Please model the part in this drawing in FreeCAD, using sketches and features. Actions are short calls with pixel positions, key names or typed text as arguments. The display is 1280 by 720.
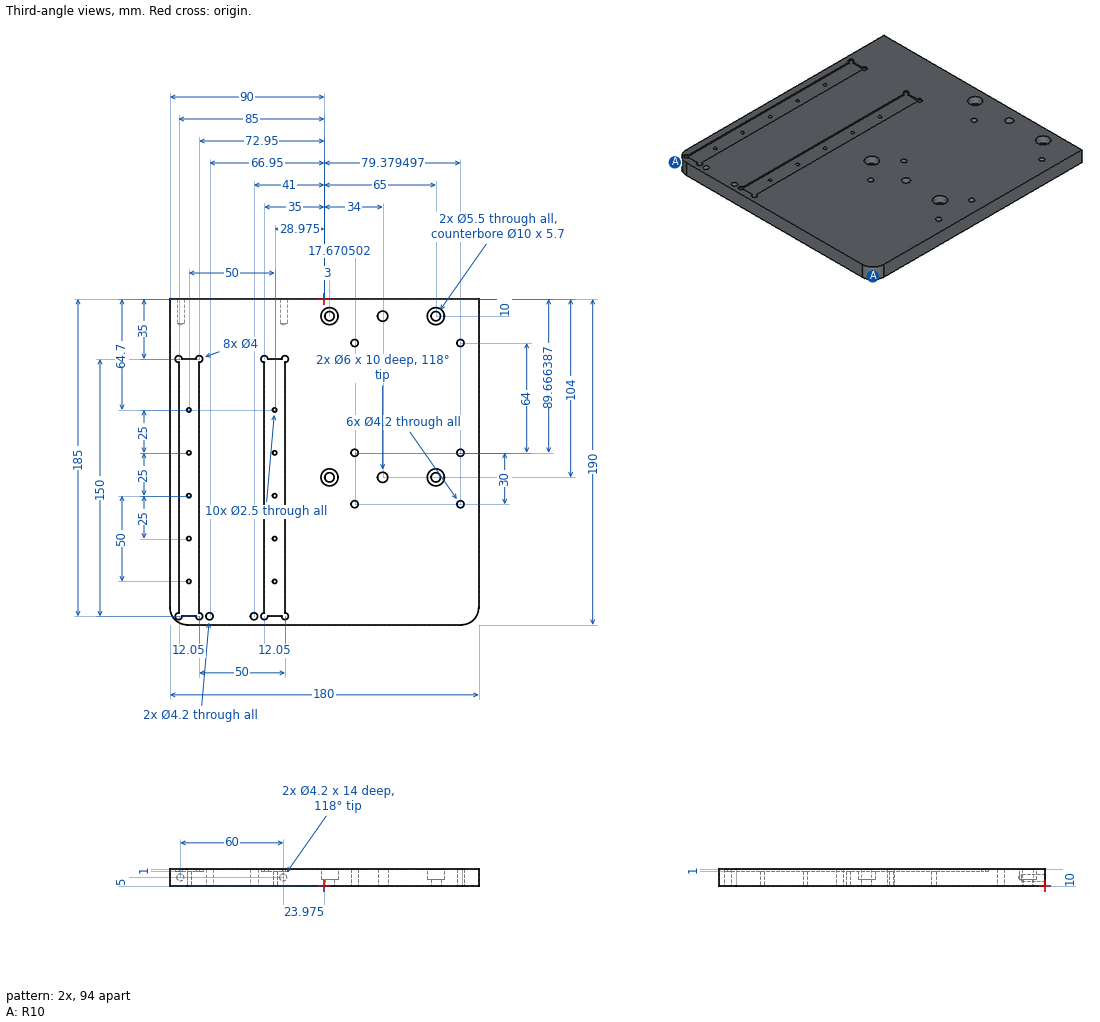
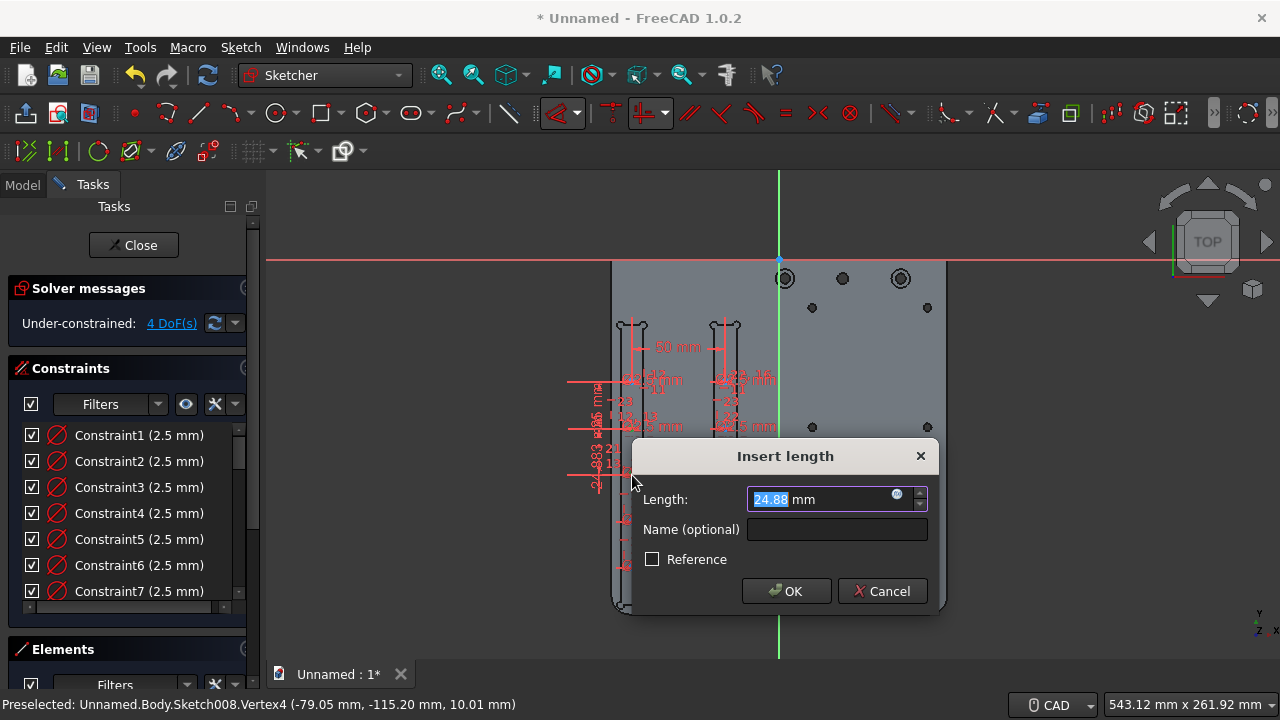
text(25)
key(Return)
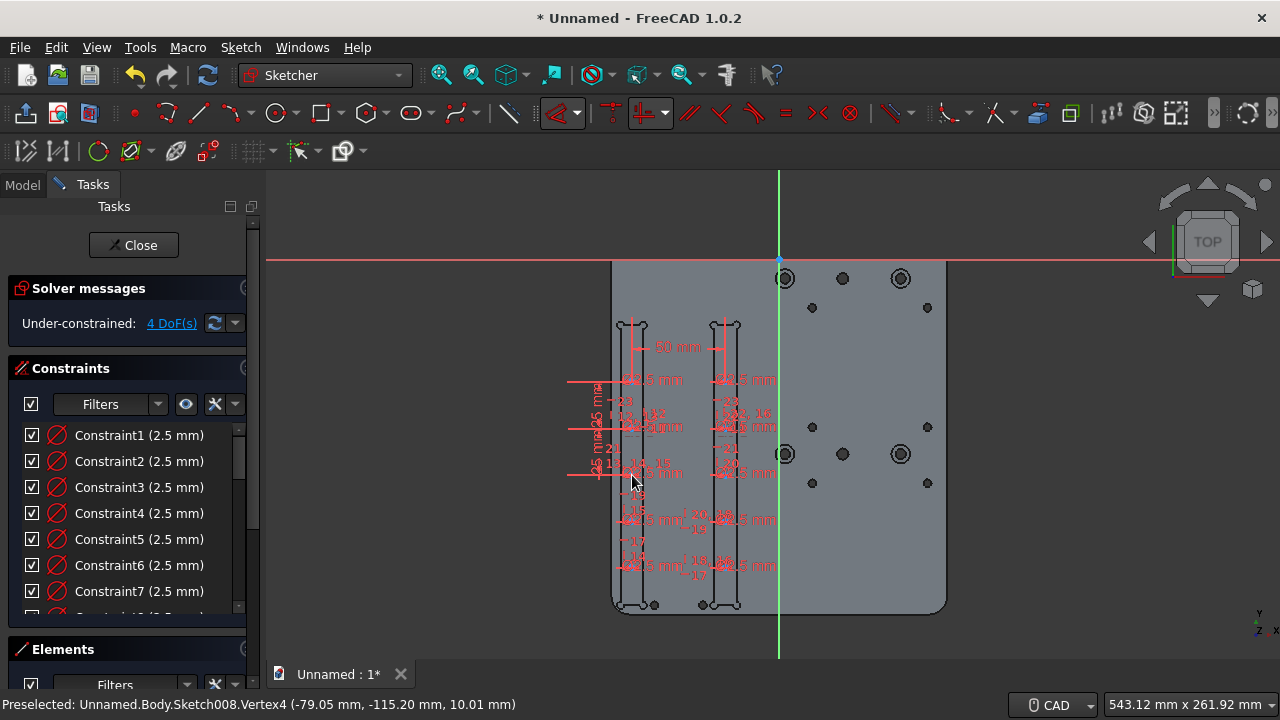
click(632, 475)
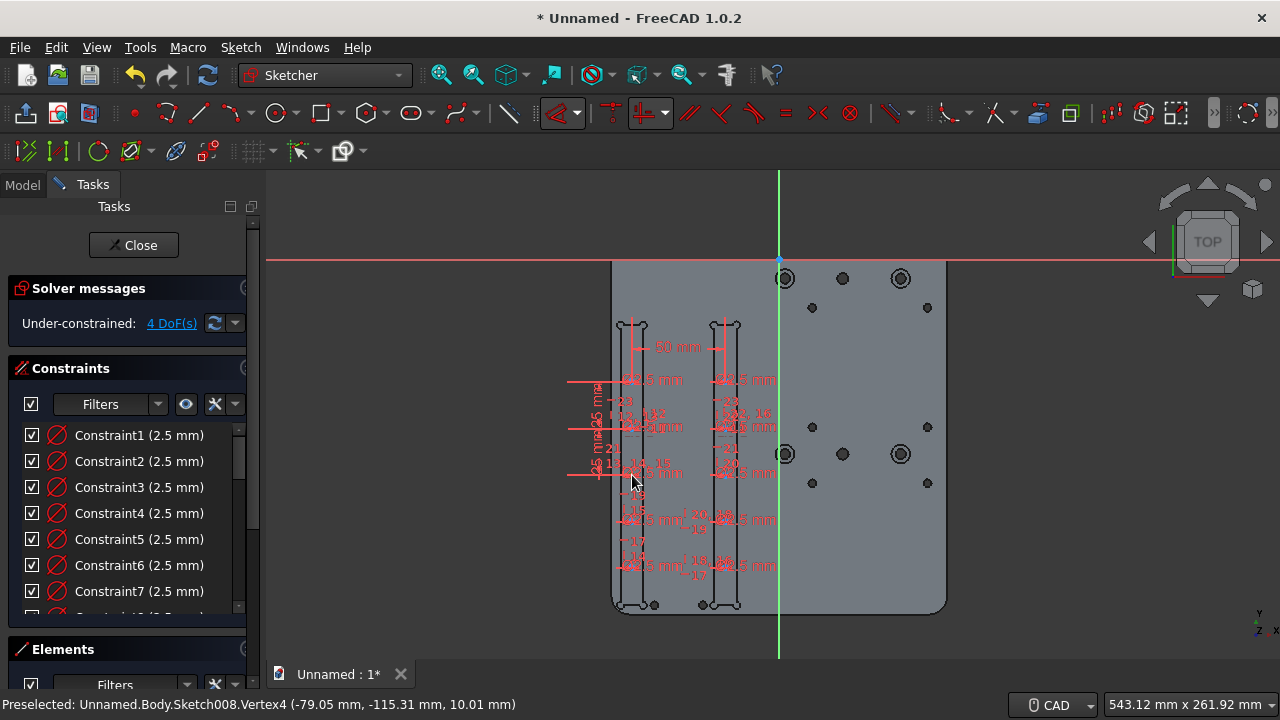
click(632, 568)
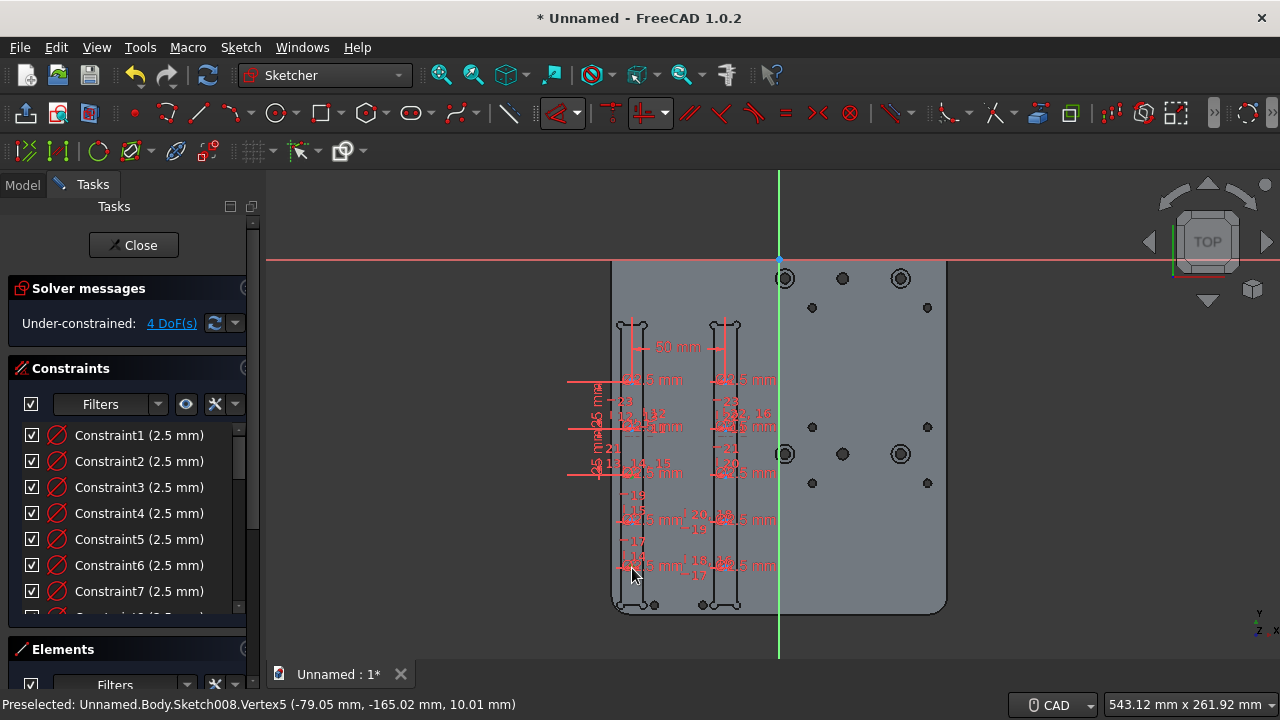
key(i)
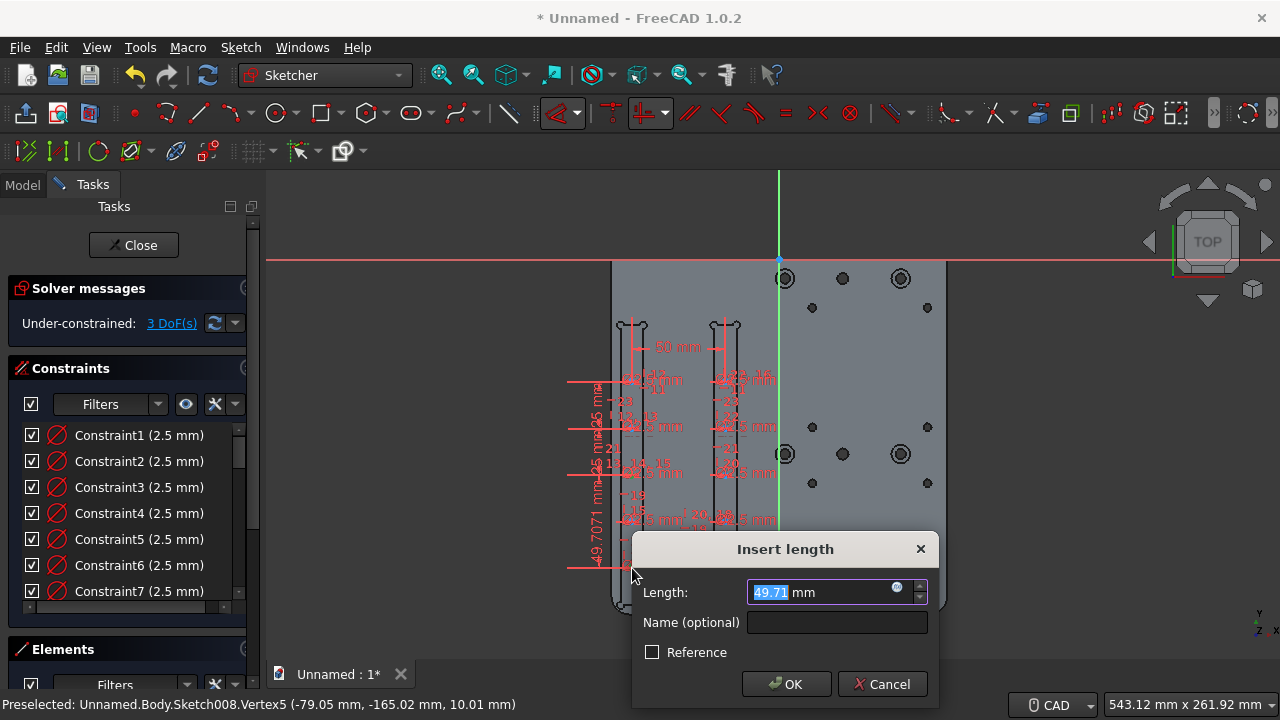
text(50)
key(Return)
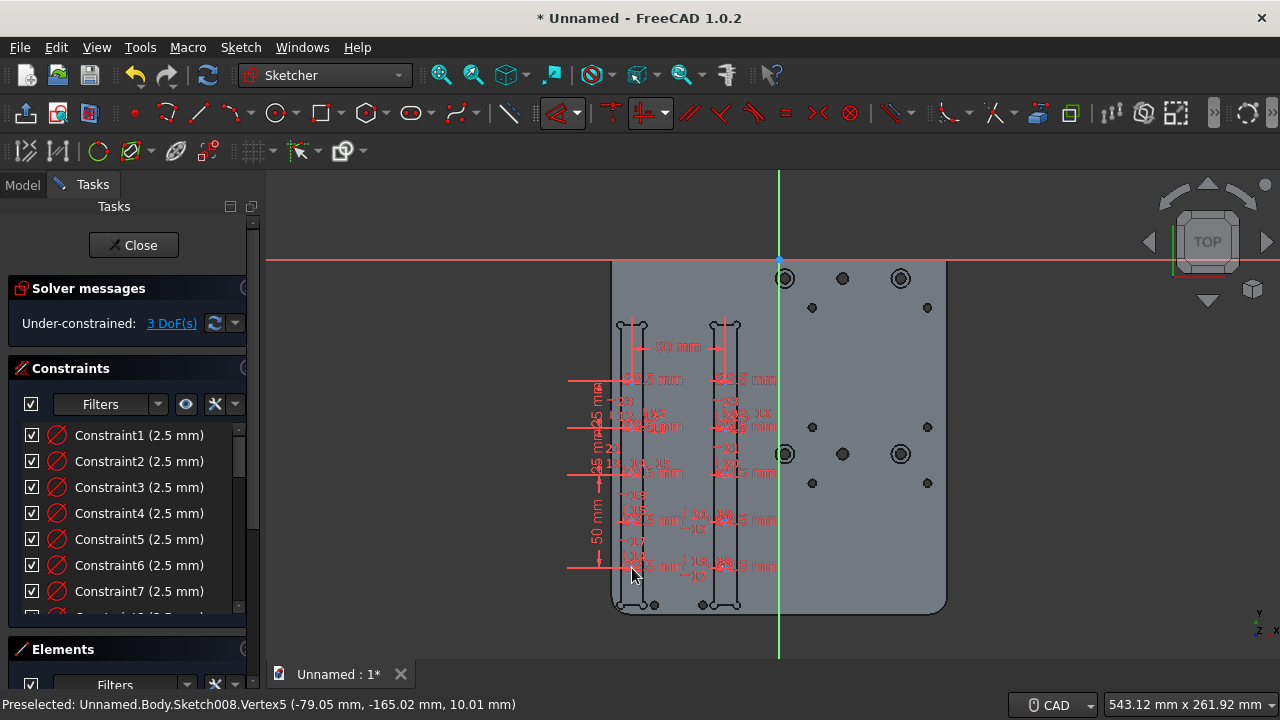
click(632, 475)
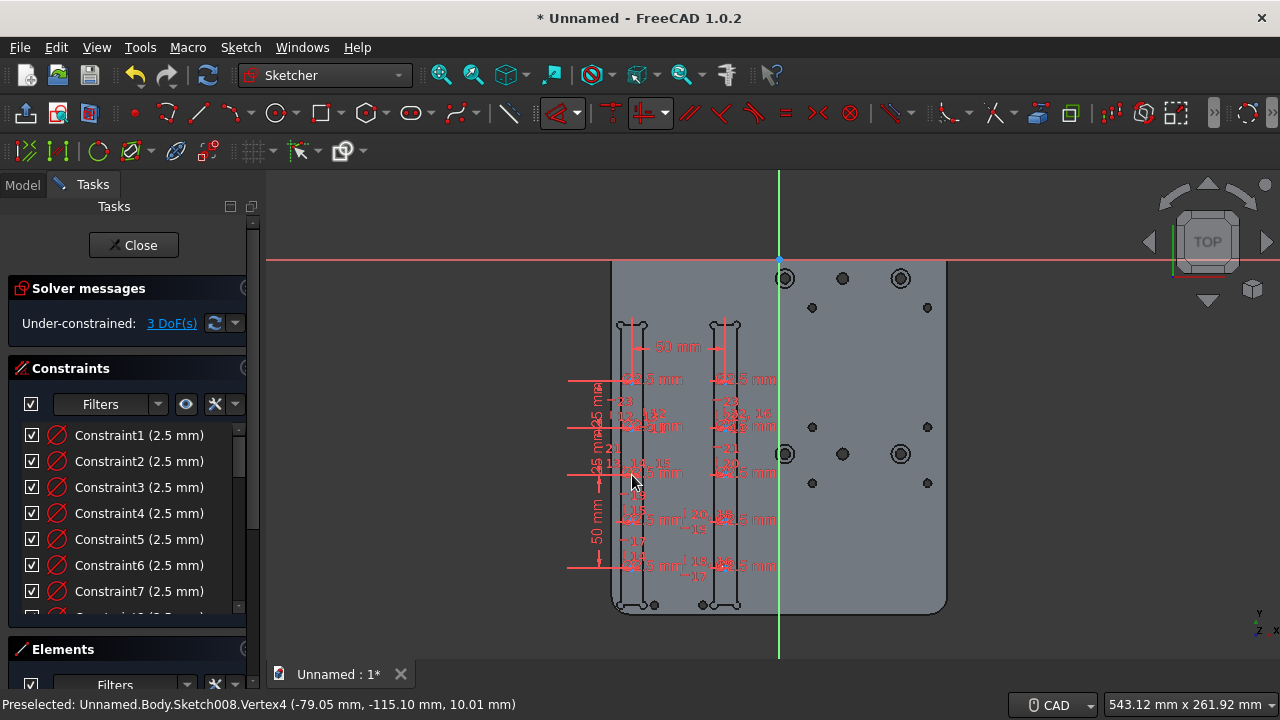
click(632, 522)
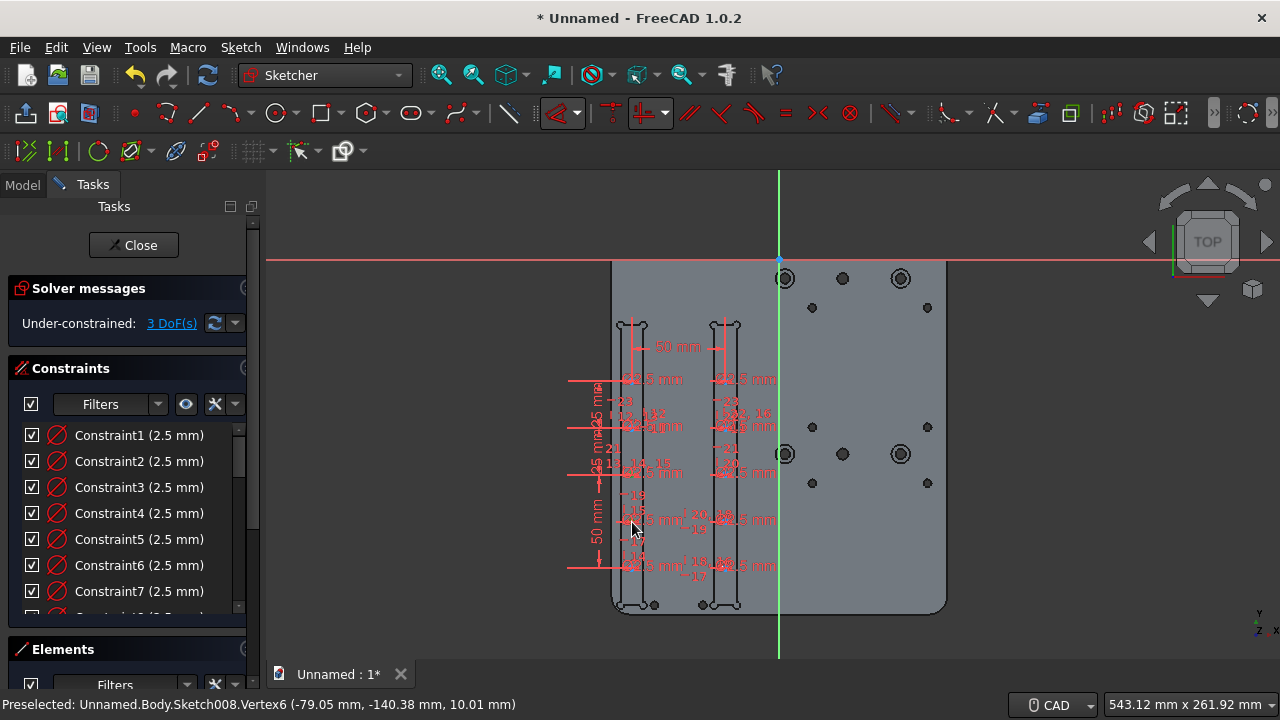
key(i)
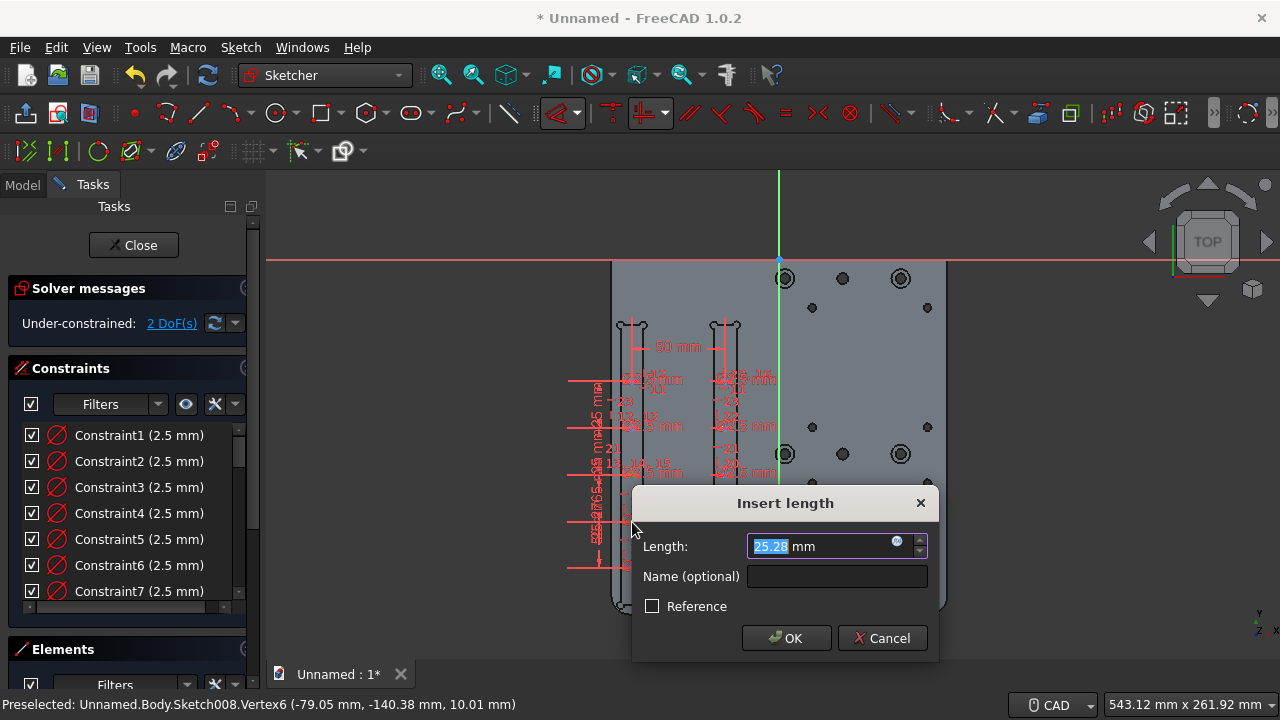
text(25)
key(Return)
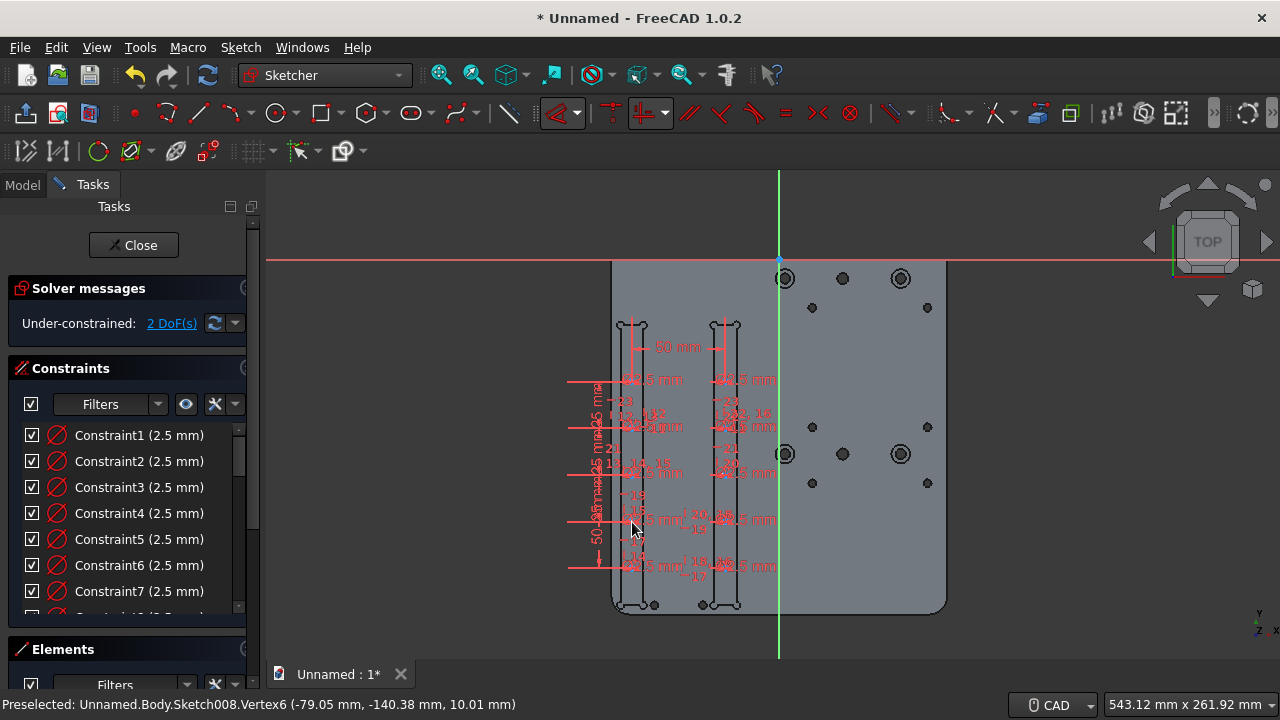
click(725, 382)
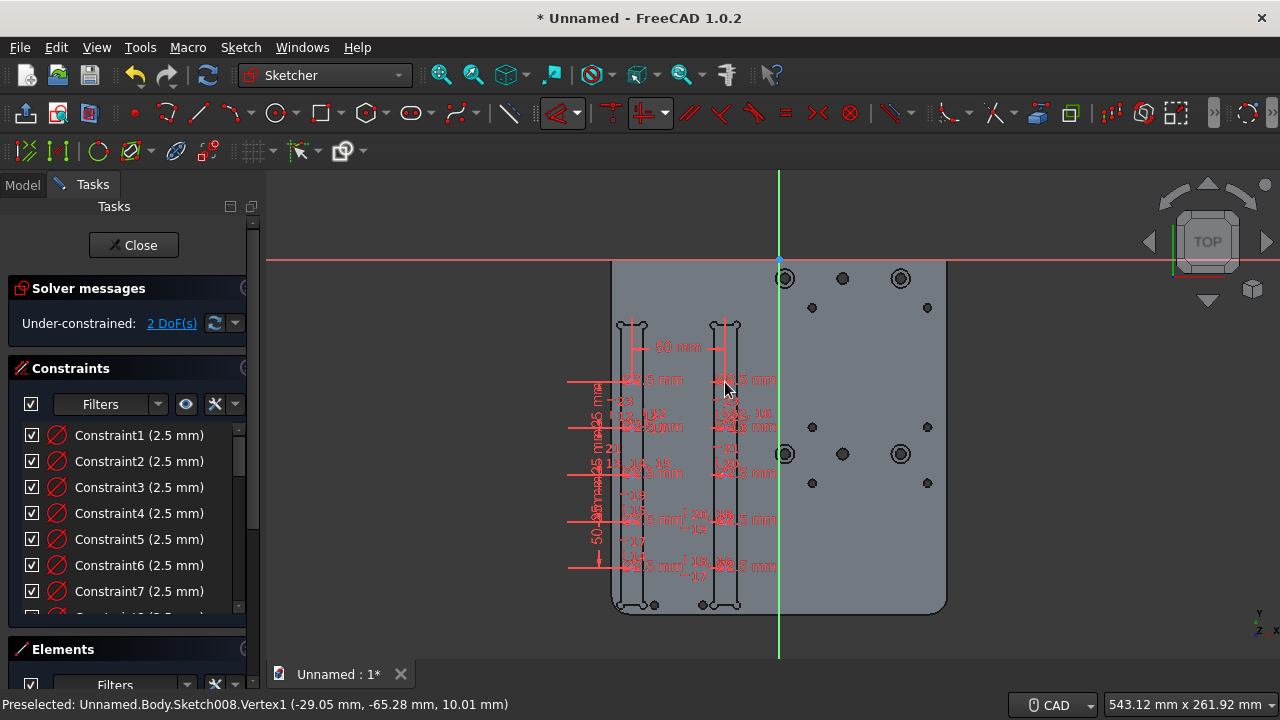
key(i)